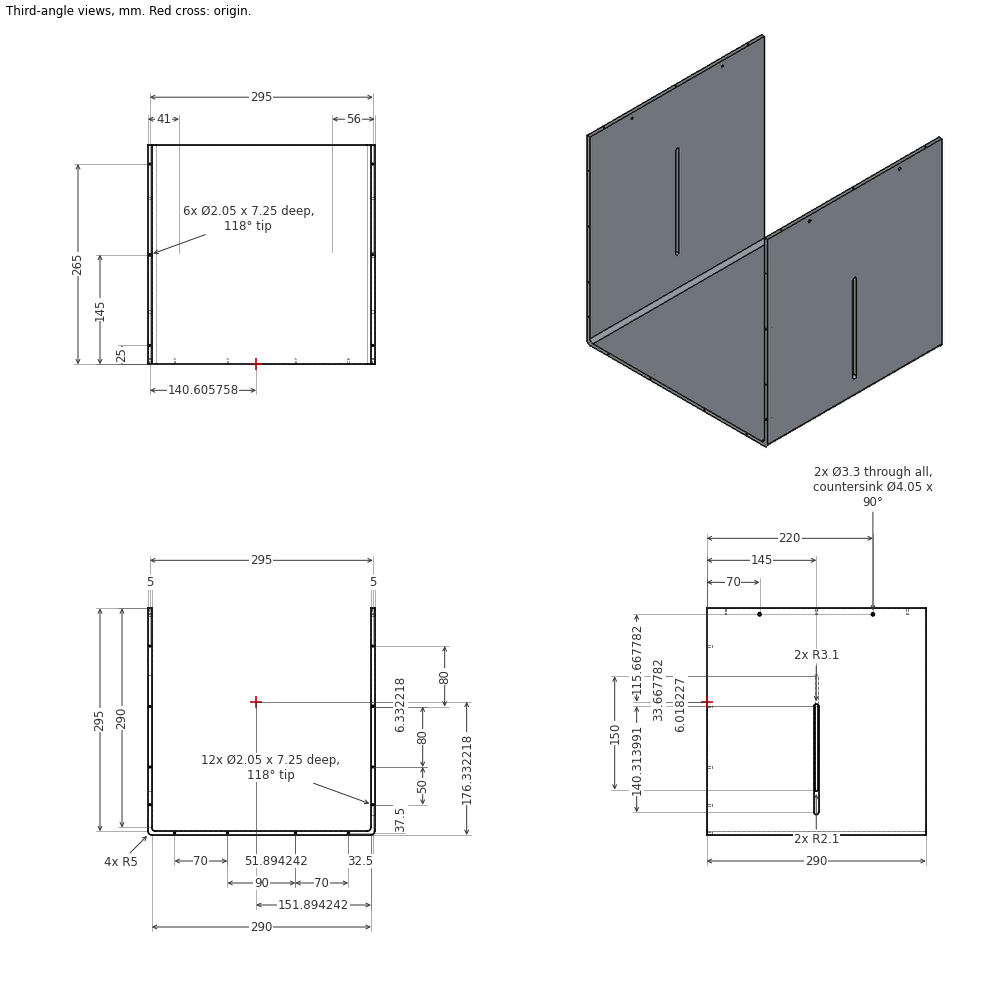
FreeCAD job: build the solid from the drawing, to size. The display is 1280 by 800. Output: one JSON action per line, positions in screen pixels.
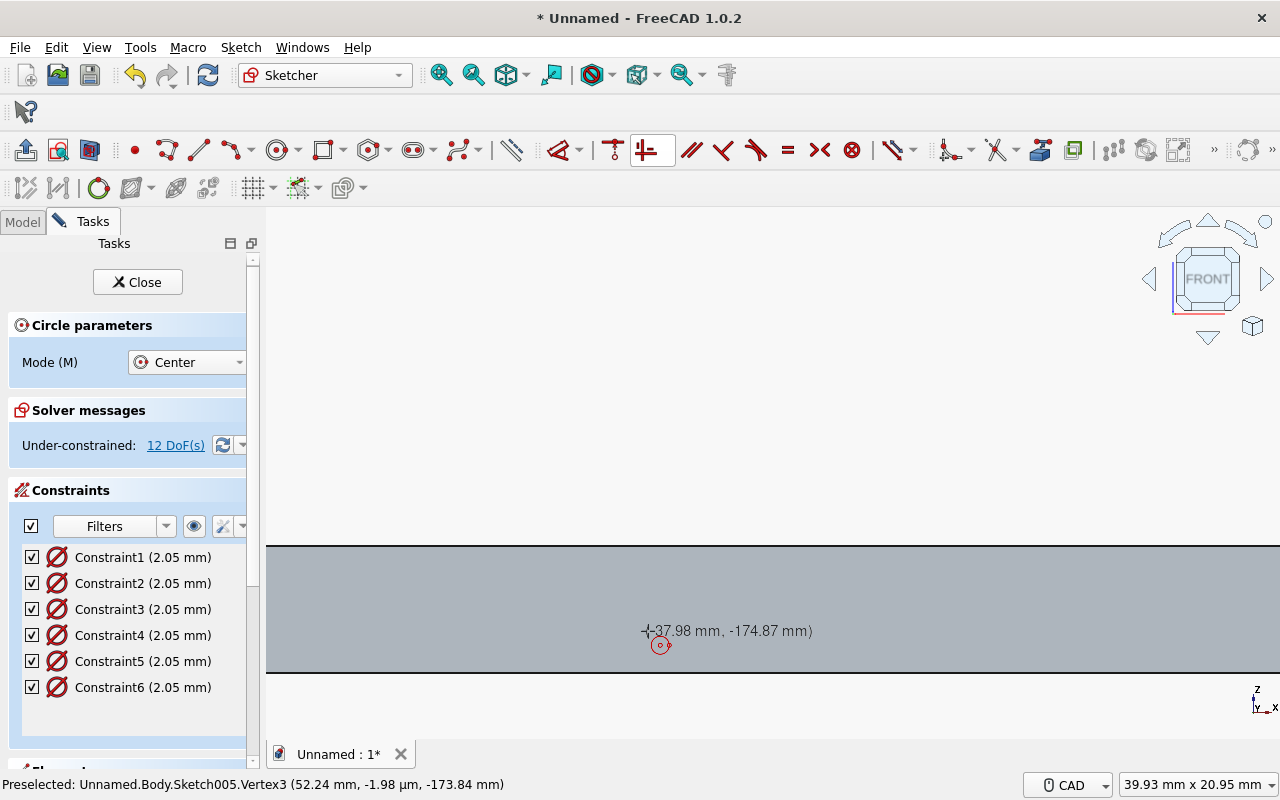
{"action": "scroll", "coordinate": [648, 631], "scroll_direction": "down", "scroll_amount": 15}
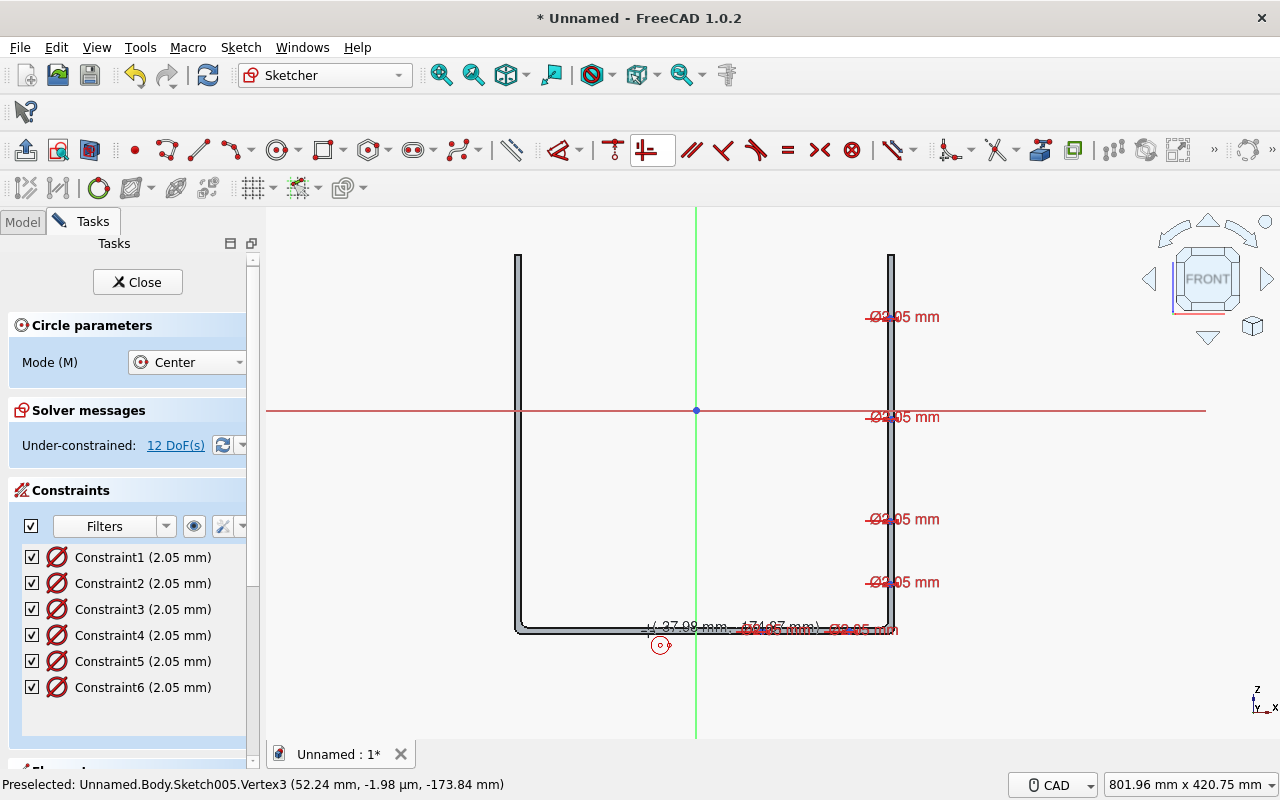
{"action": "left_click", "coordinate": [648, 631]}
{"action": "mouse_move", "coordinate": [649, 630]}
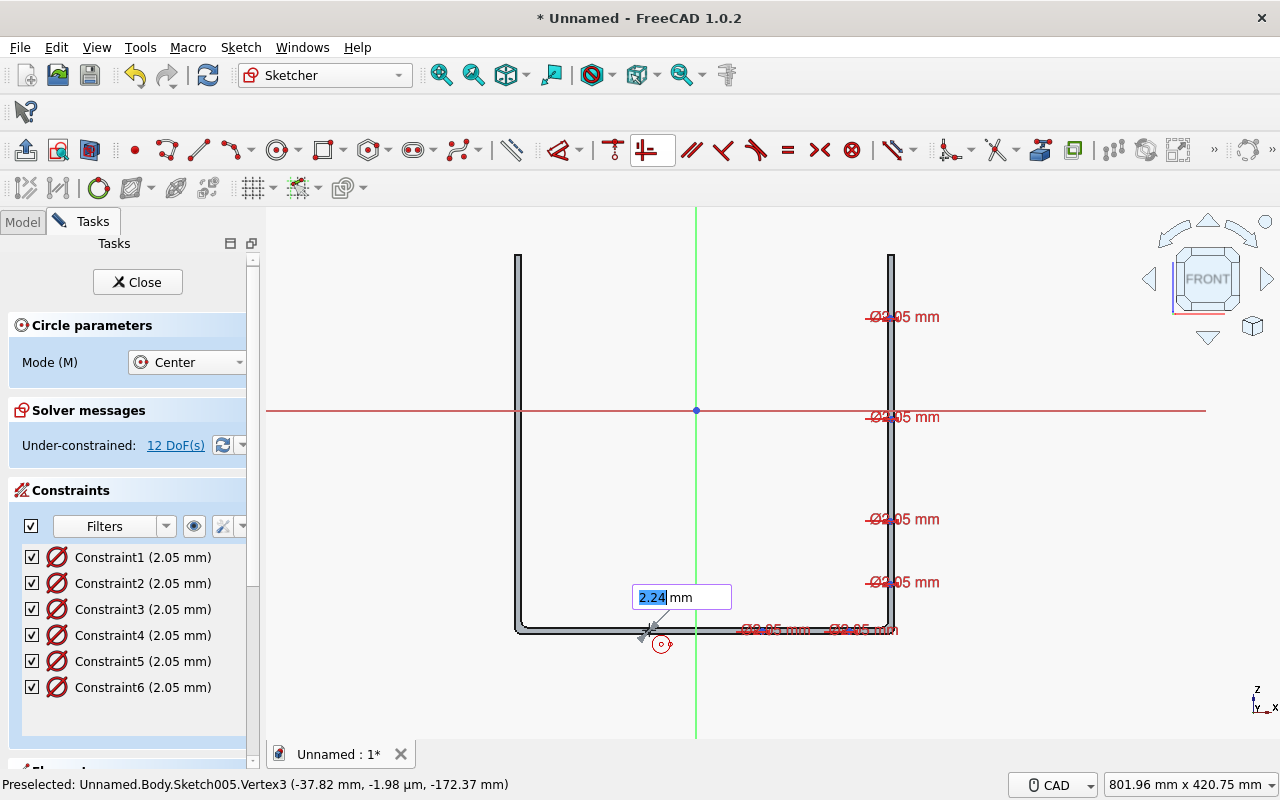
{"action": "type", "text": "2.05"}
{"action": "key", "text": "Return"}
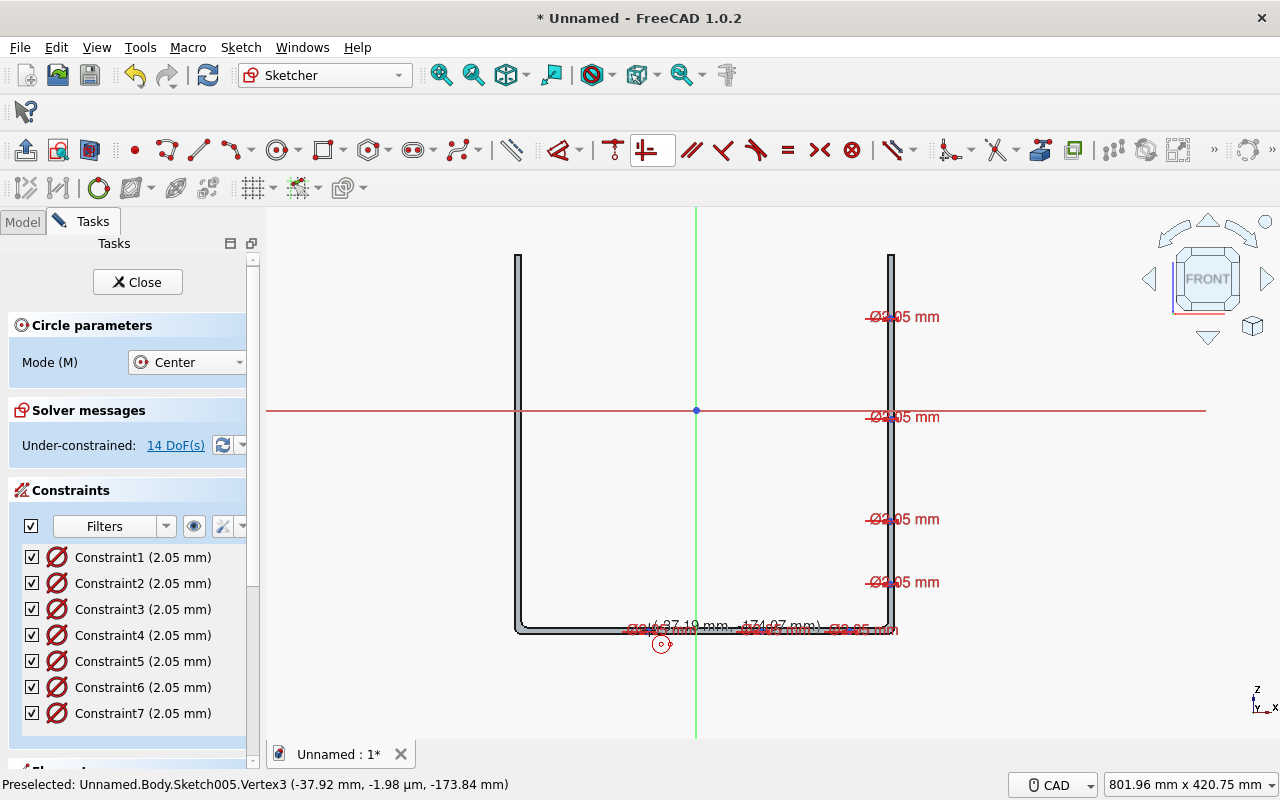
{"action": "scroll", "coordinate": [559, 631], "scroll_direction": "up", "scroll_amount": 15}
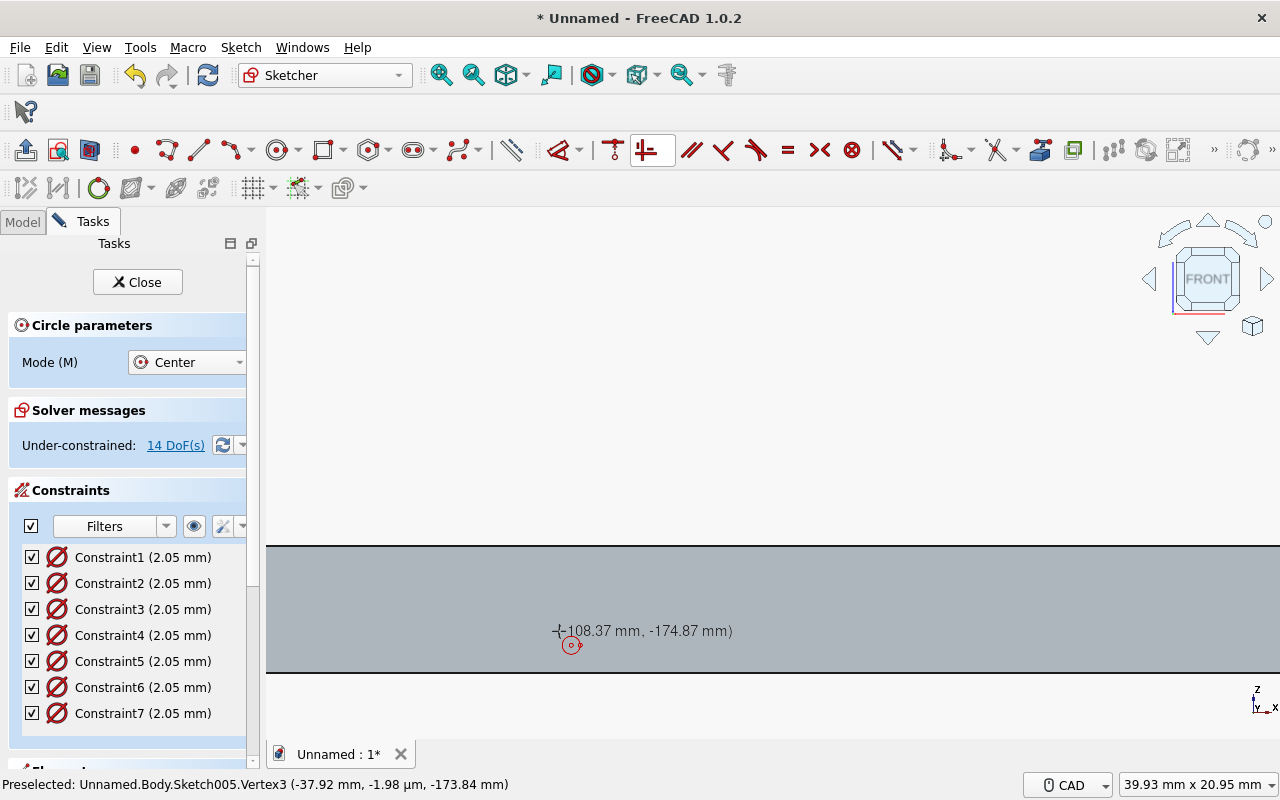
{"action": "scroll", "coordinate": [559, 631], "scroll_direction": "down", "scroll_amount": 15}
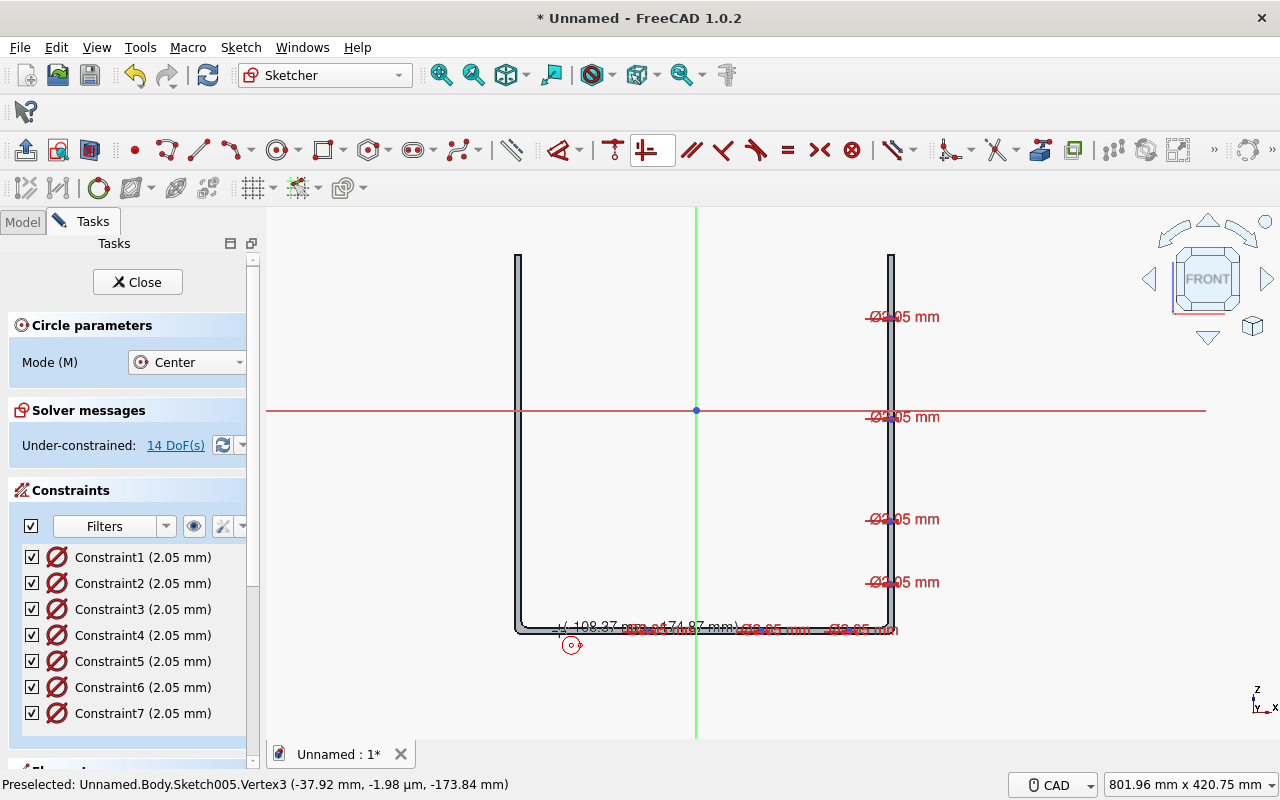
{"action": "left_click", "coordinate": [559, 631]}
{"action": "mouse_move", "coordinate": [560, 630]}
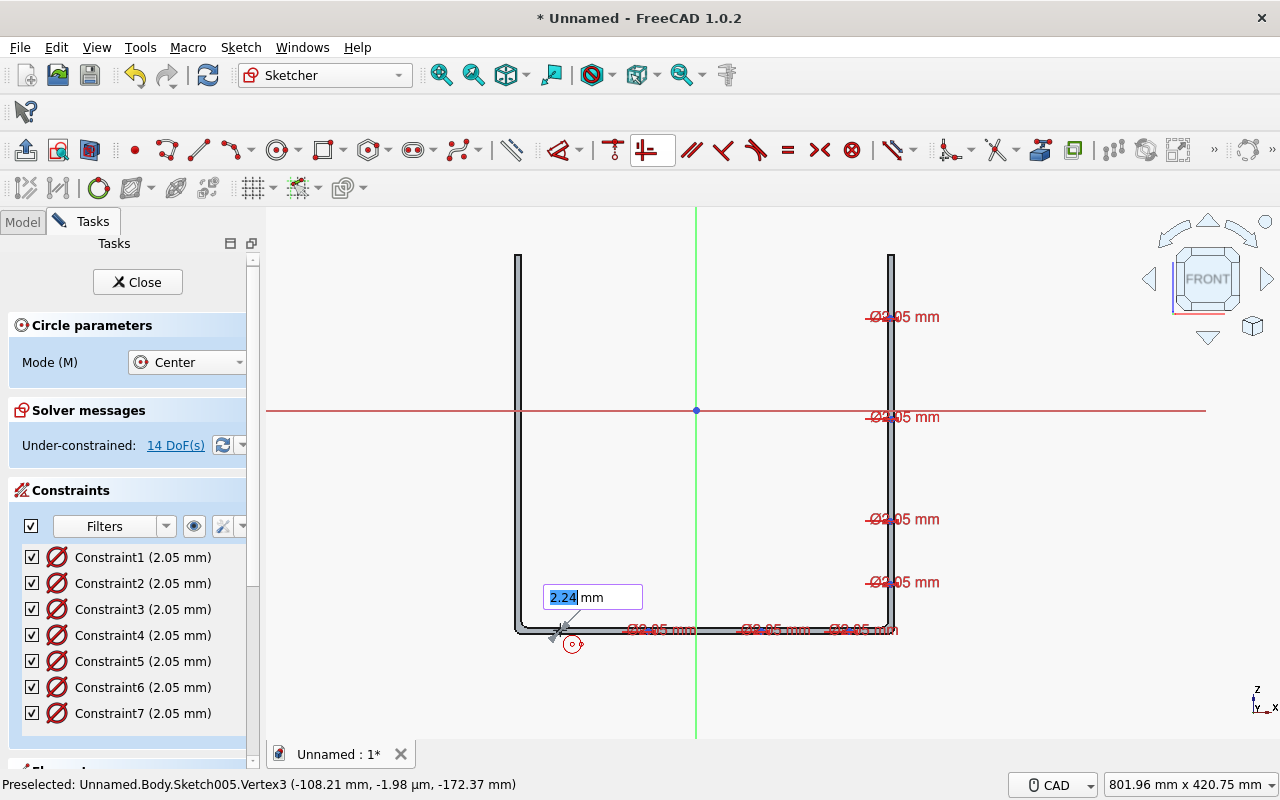
{"action": "type", "text": "2.05"}
{"action": "key", "text": "Return"}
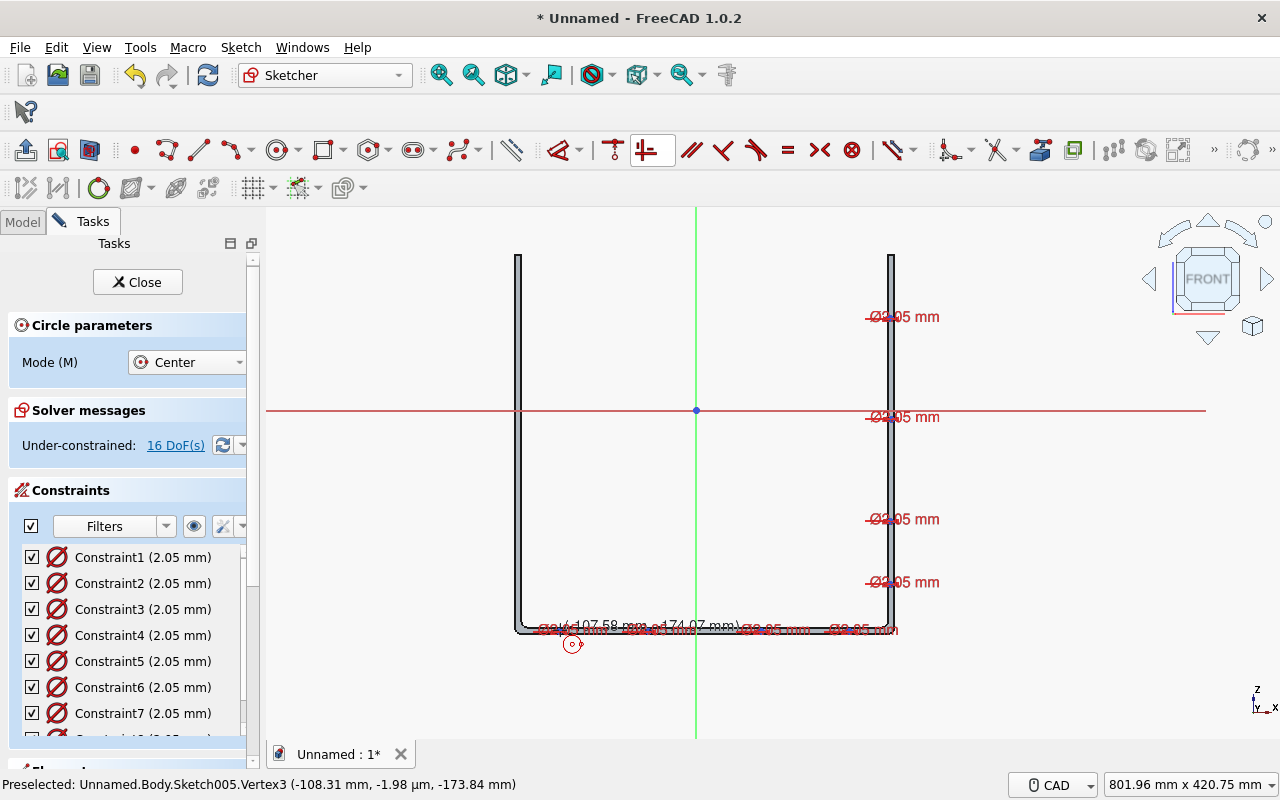
{"action": "scroll", "coordinate": [518, 318], "scroll_direction": "up", "scroll_amount": 15}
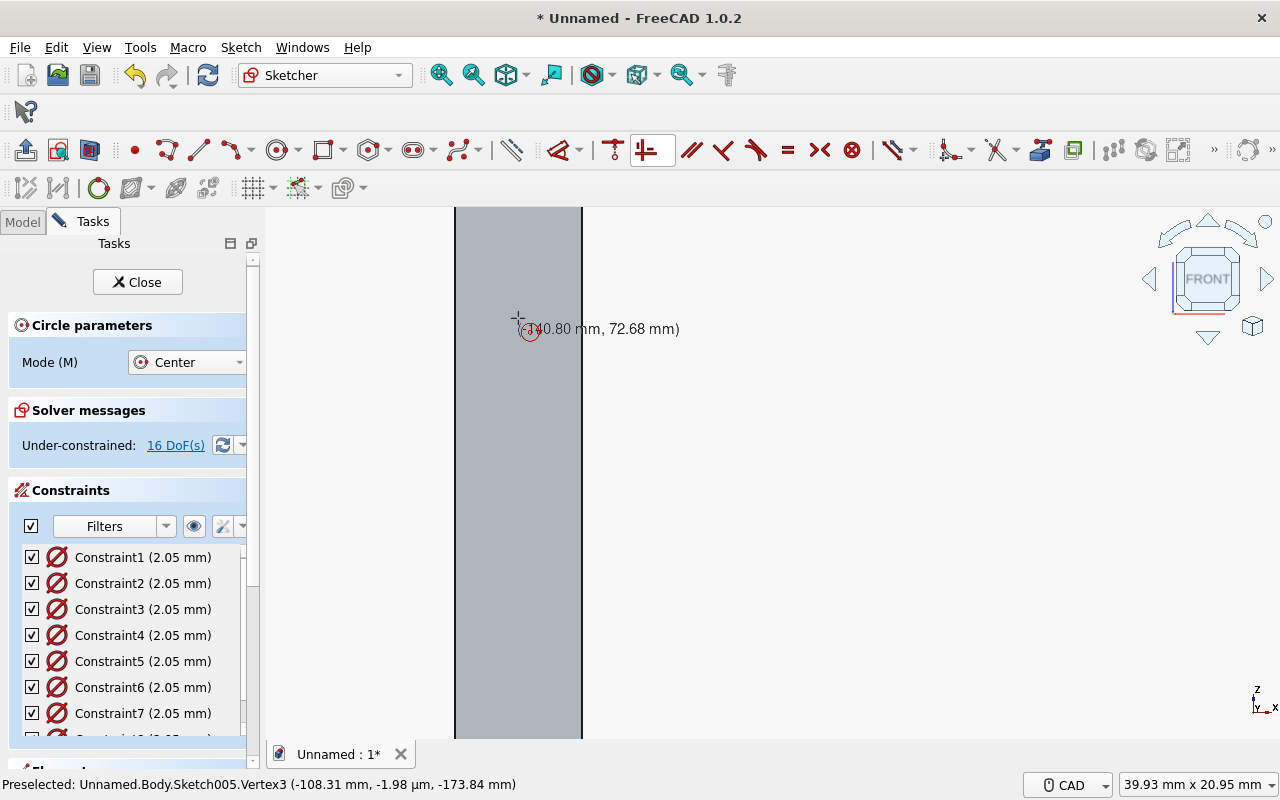
{"action": "scroll", "coordinate": [518, 317], "scroll_direction": "down", "scroll_amount": 15}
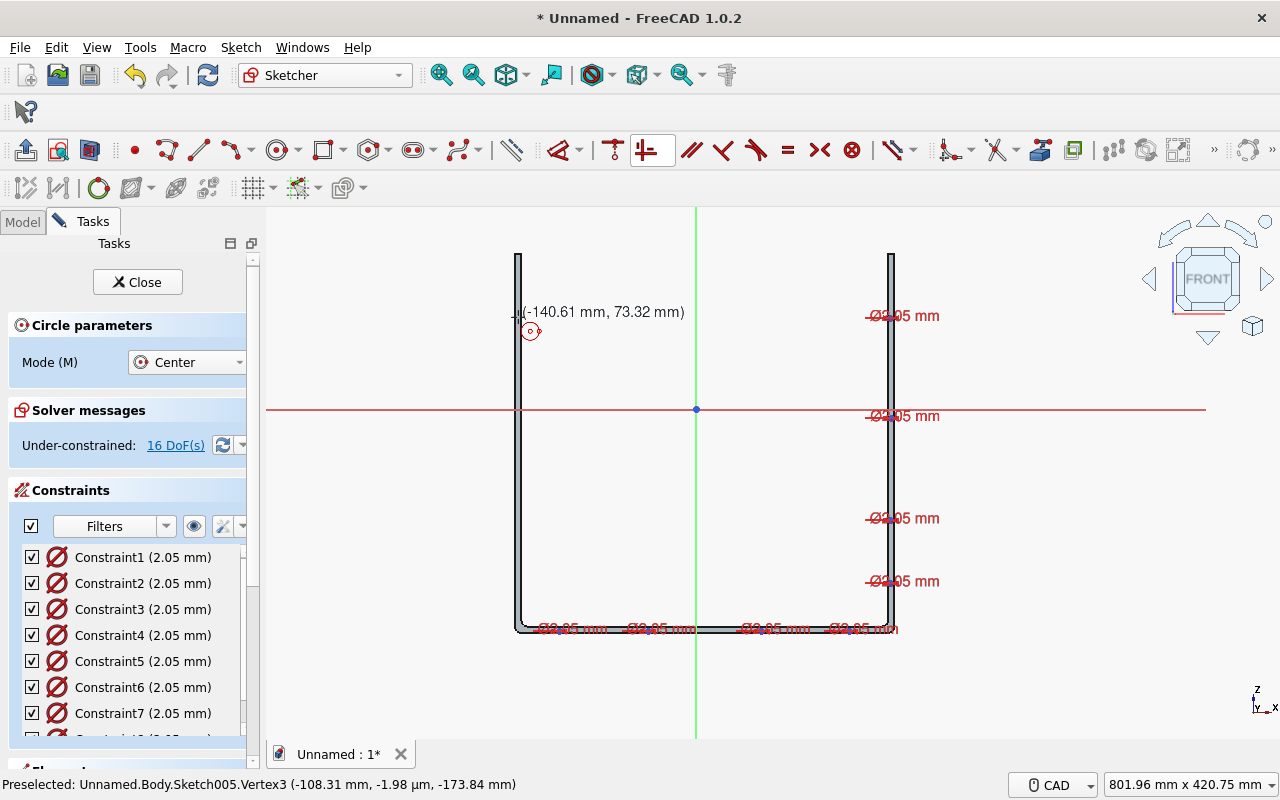
{"action": "left_click", "coordinate": [518, 317]}
{"action": "mouse_move", "coordinate": [519, 316]}